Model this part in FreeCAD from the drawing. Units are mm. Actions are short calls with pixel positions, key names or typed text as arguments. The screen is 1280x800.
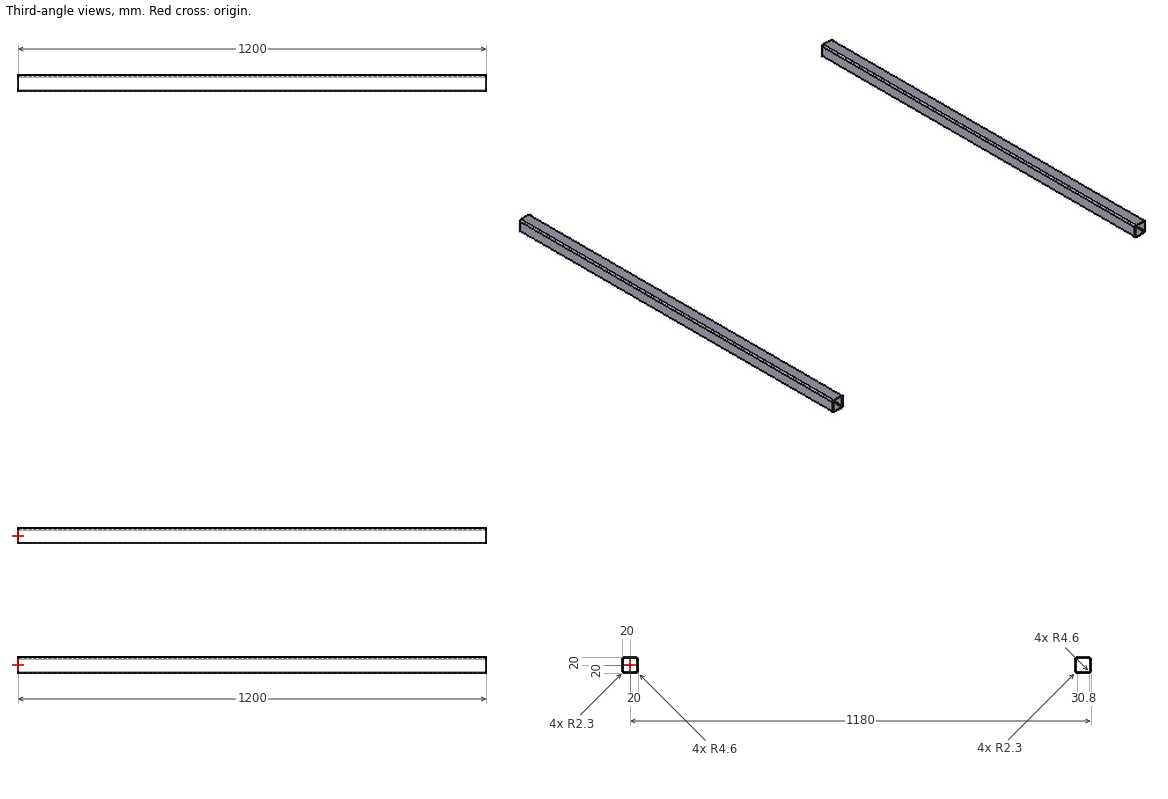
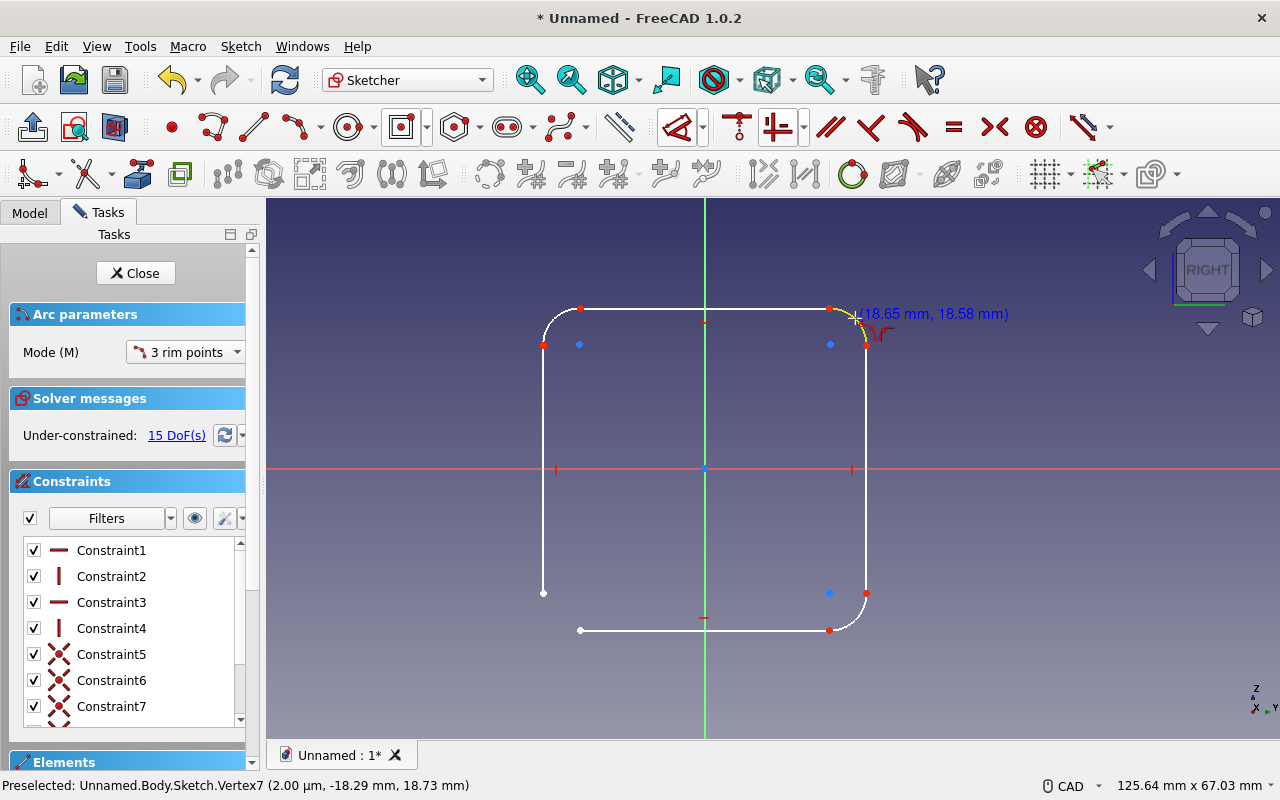
click(543, 594)
click(580, 631)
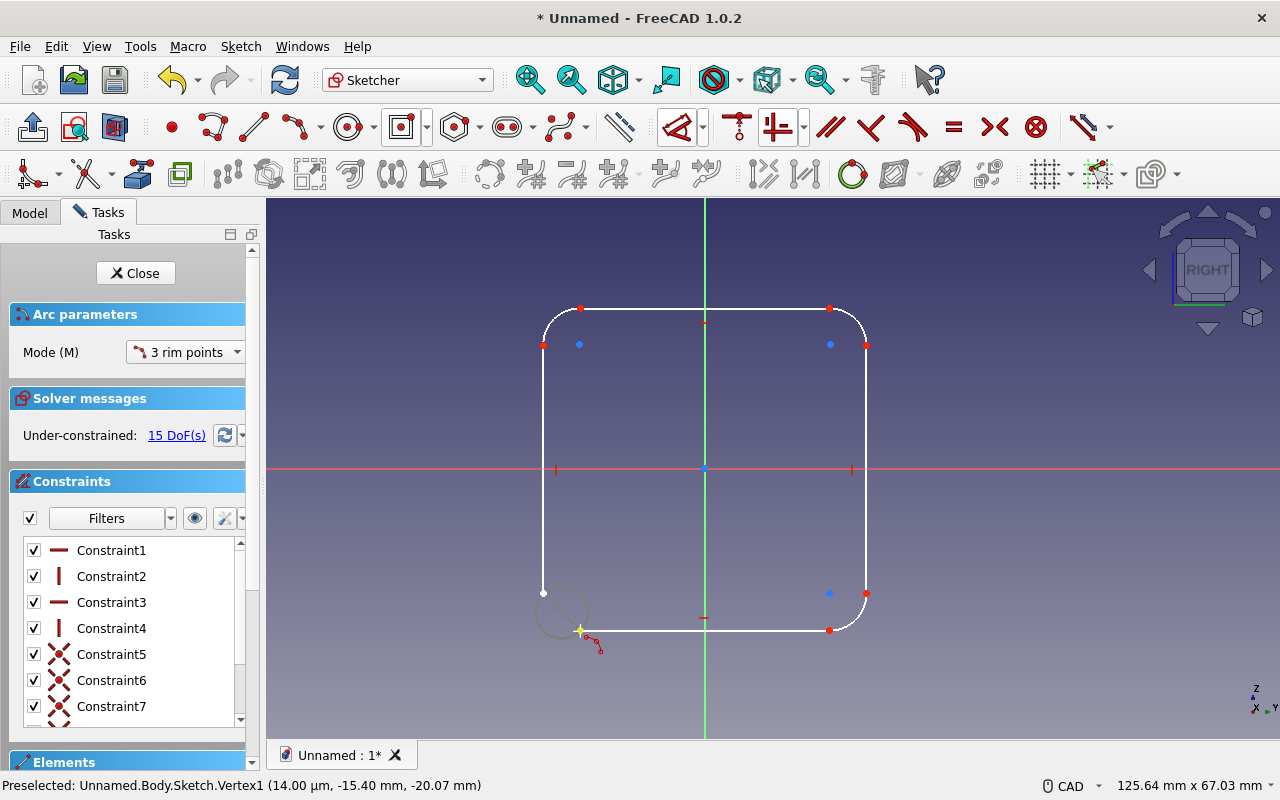
scroll(554, 619, up, 2)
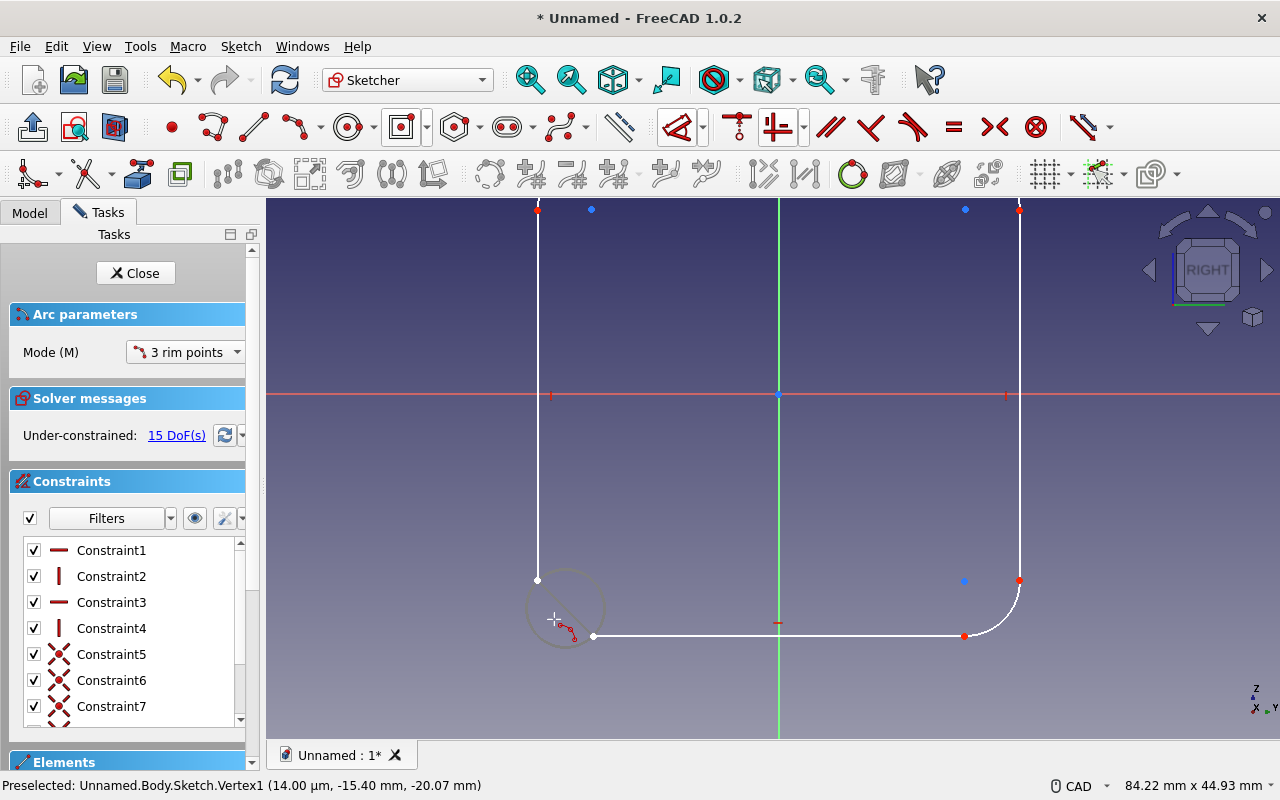
click(554, 619)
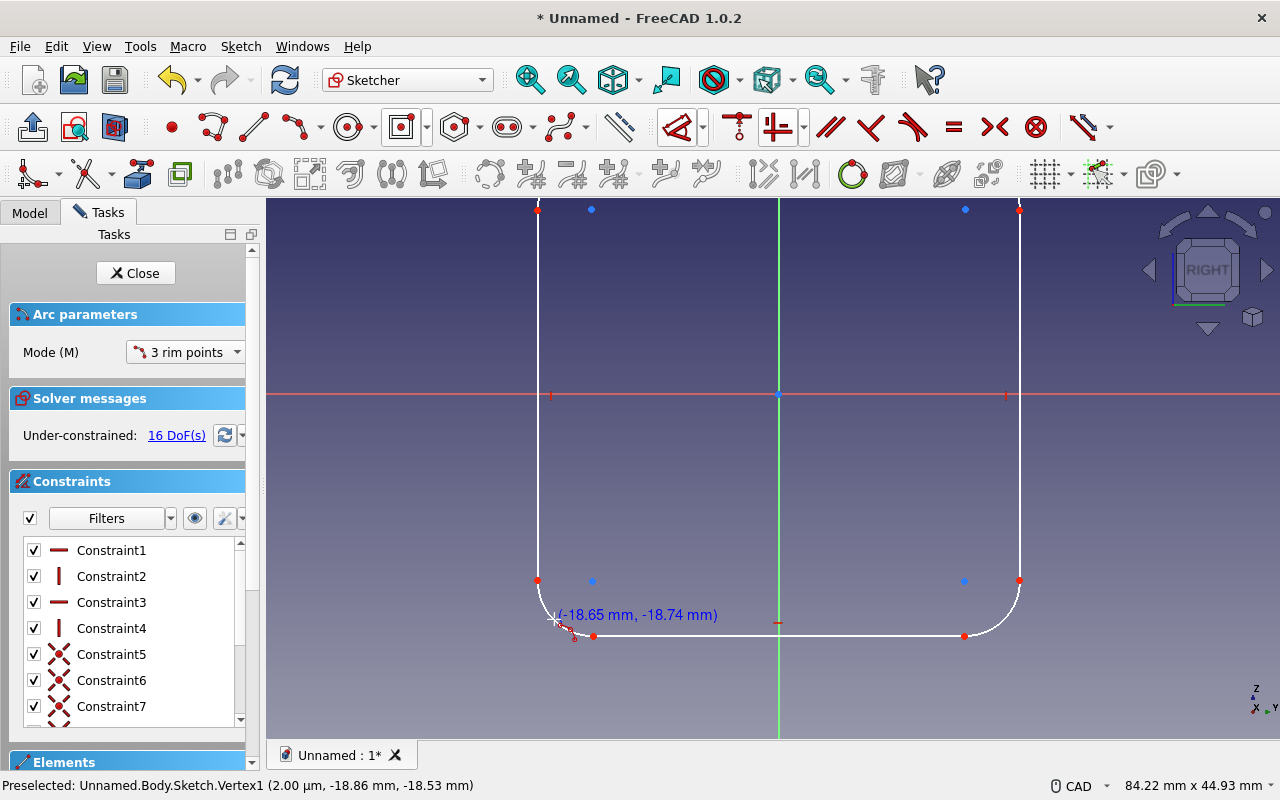
key(g)
key(l)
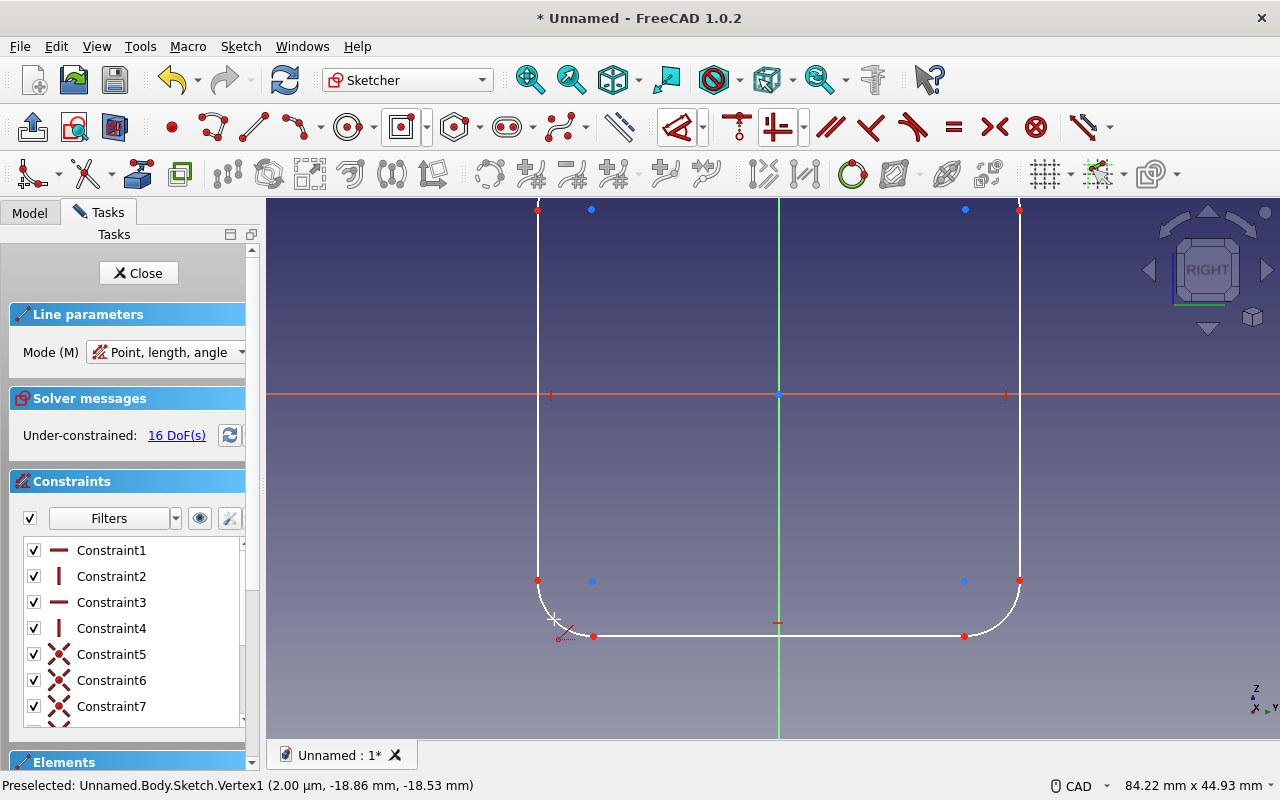
click(964, 607)
click(593, 607)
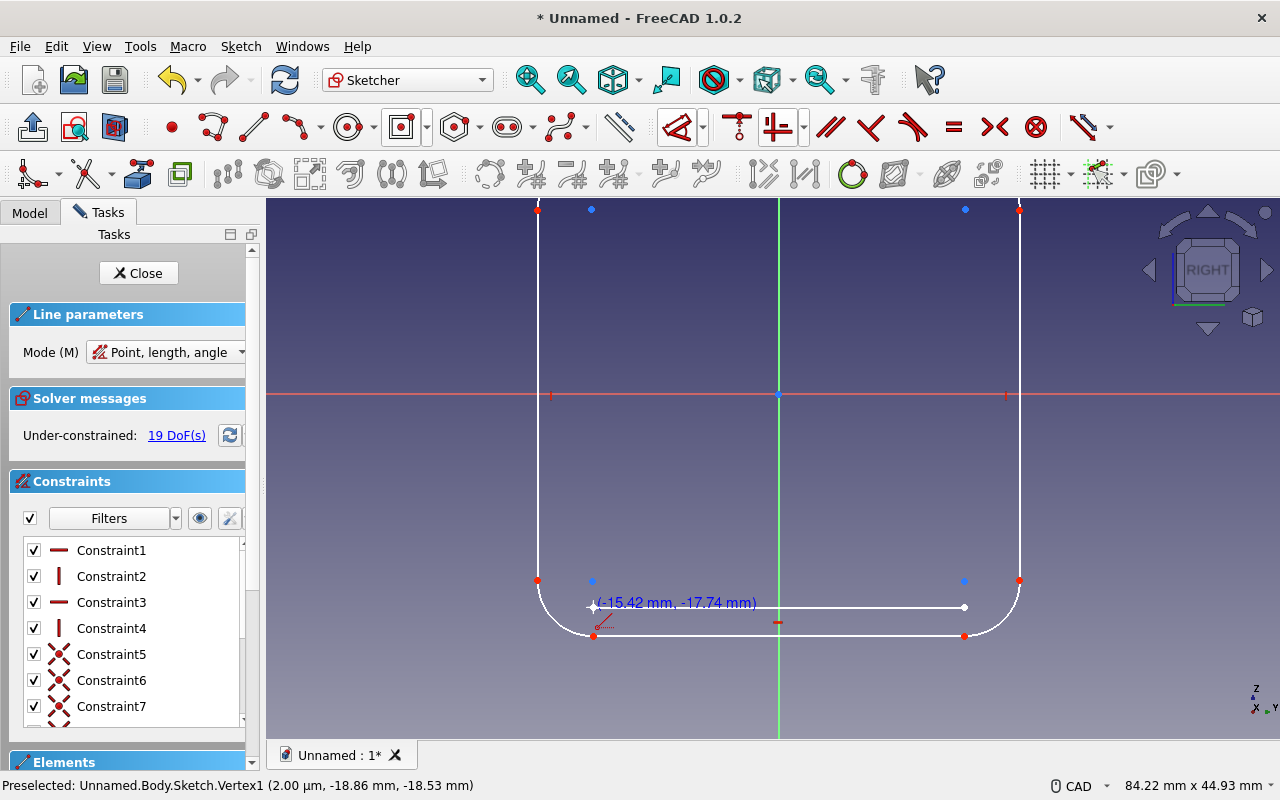
click(565, 580)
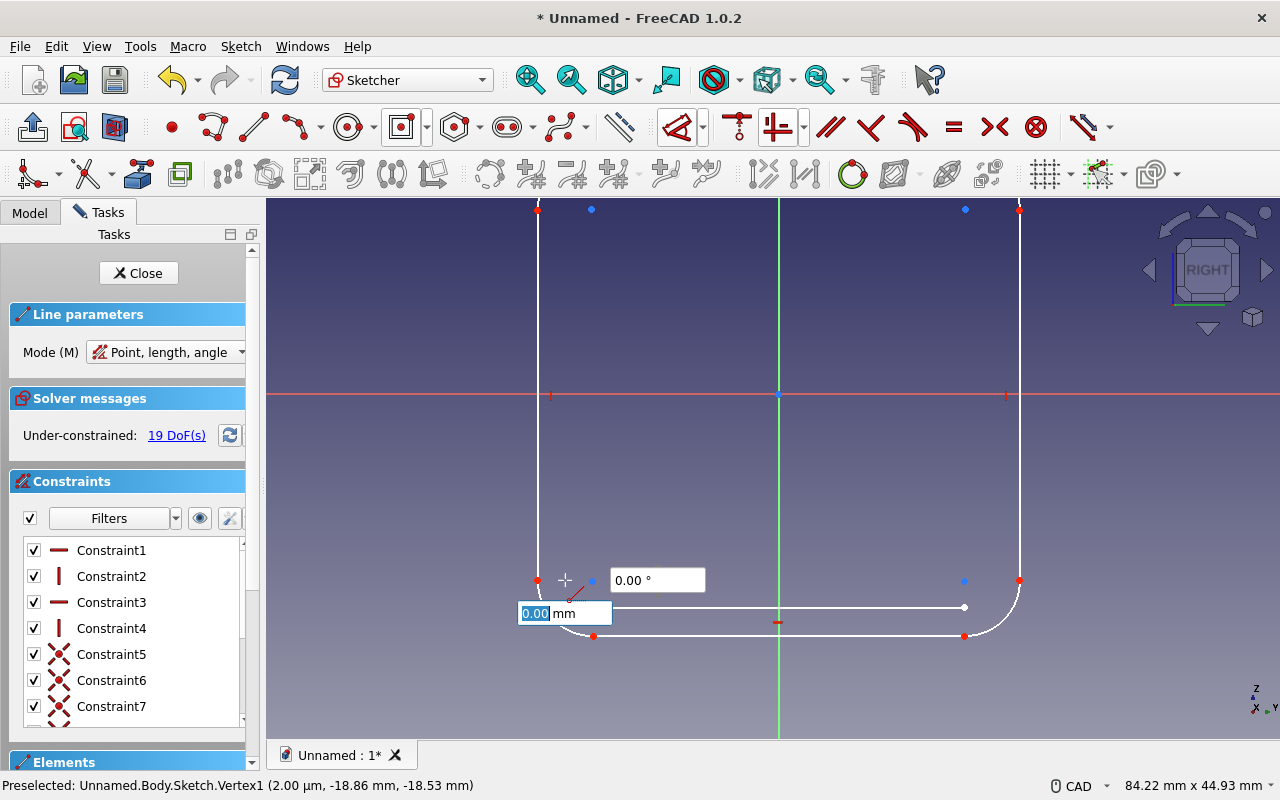
scroll(554, 619, down, 2)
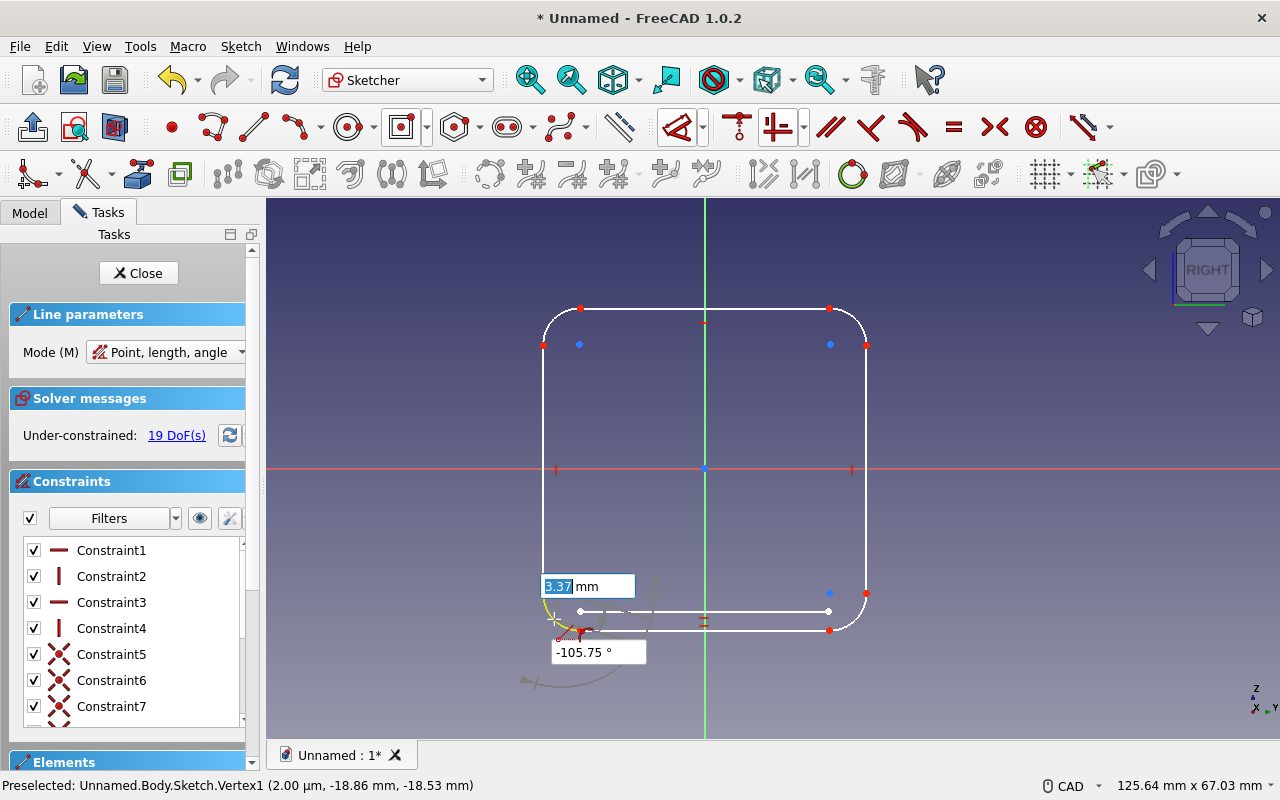
click(561, 344)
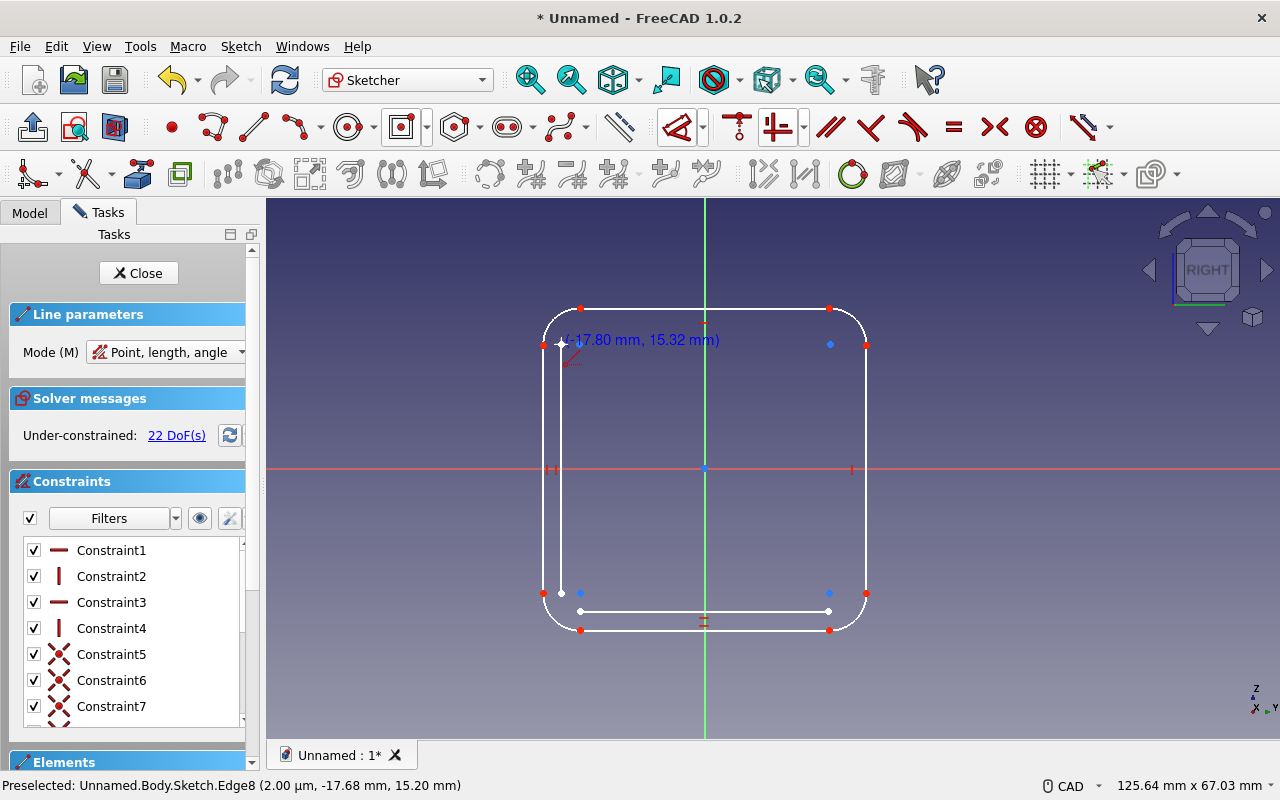
click(580, 326)
click(829, 326)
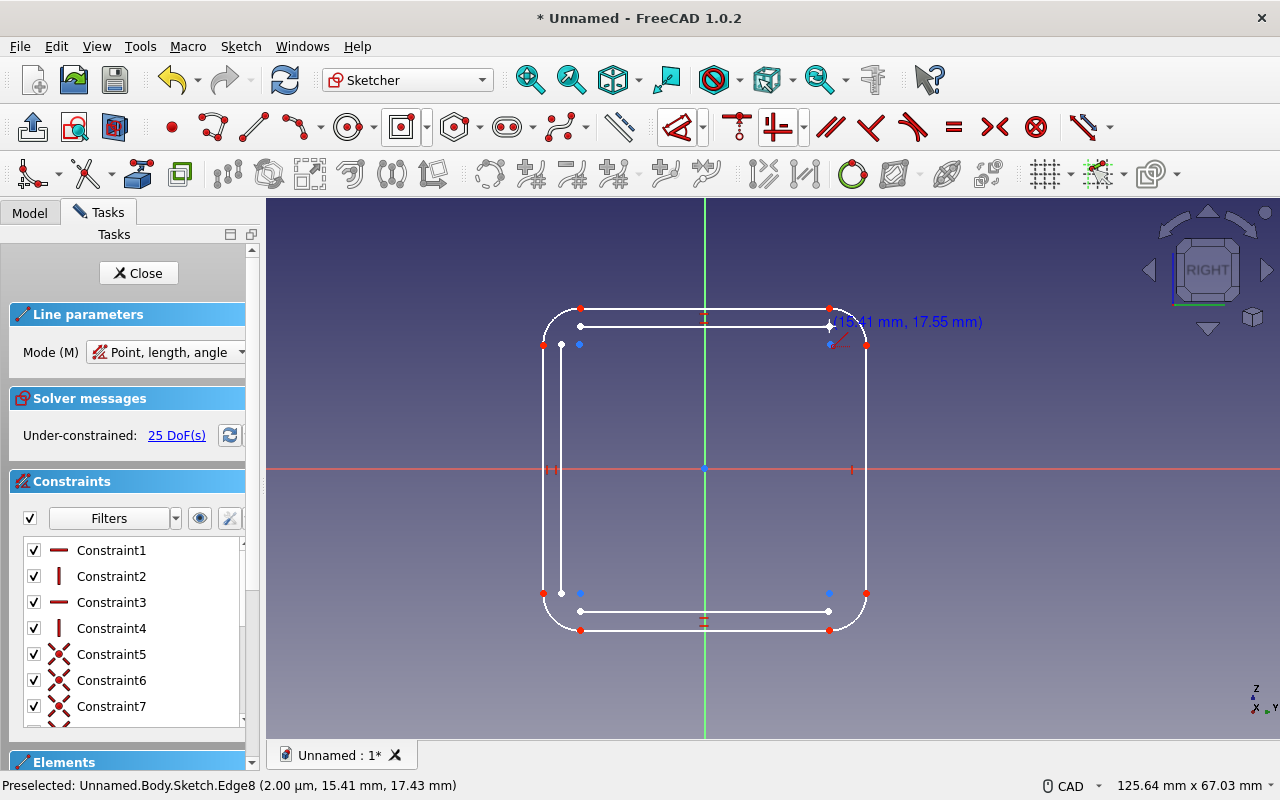
click(848, 344)
click(848, 593)